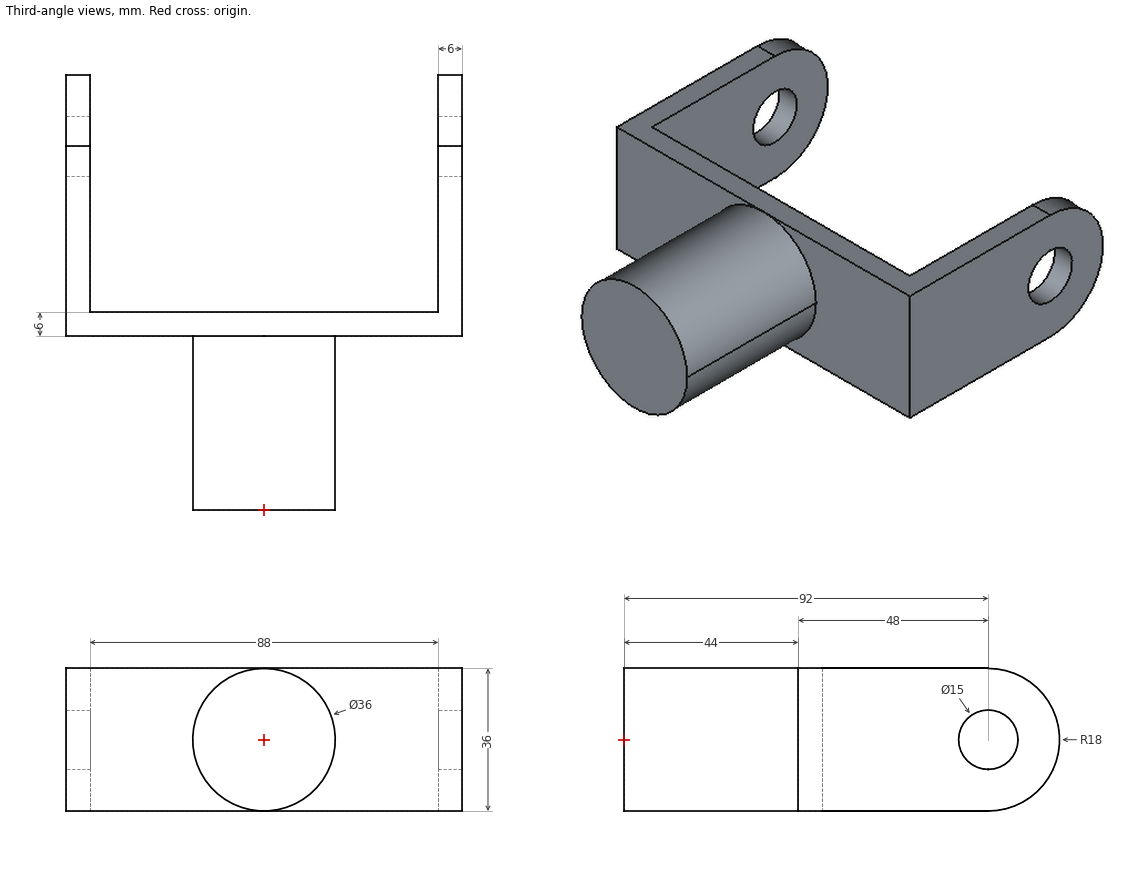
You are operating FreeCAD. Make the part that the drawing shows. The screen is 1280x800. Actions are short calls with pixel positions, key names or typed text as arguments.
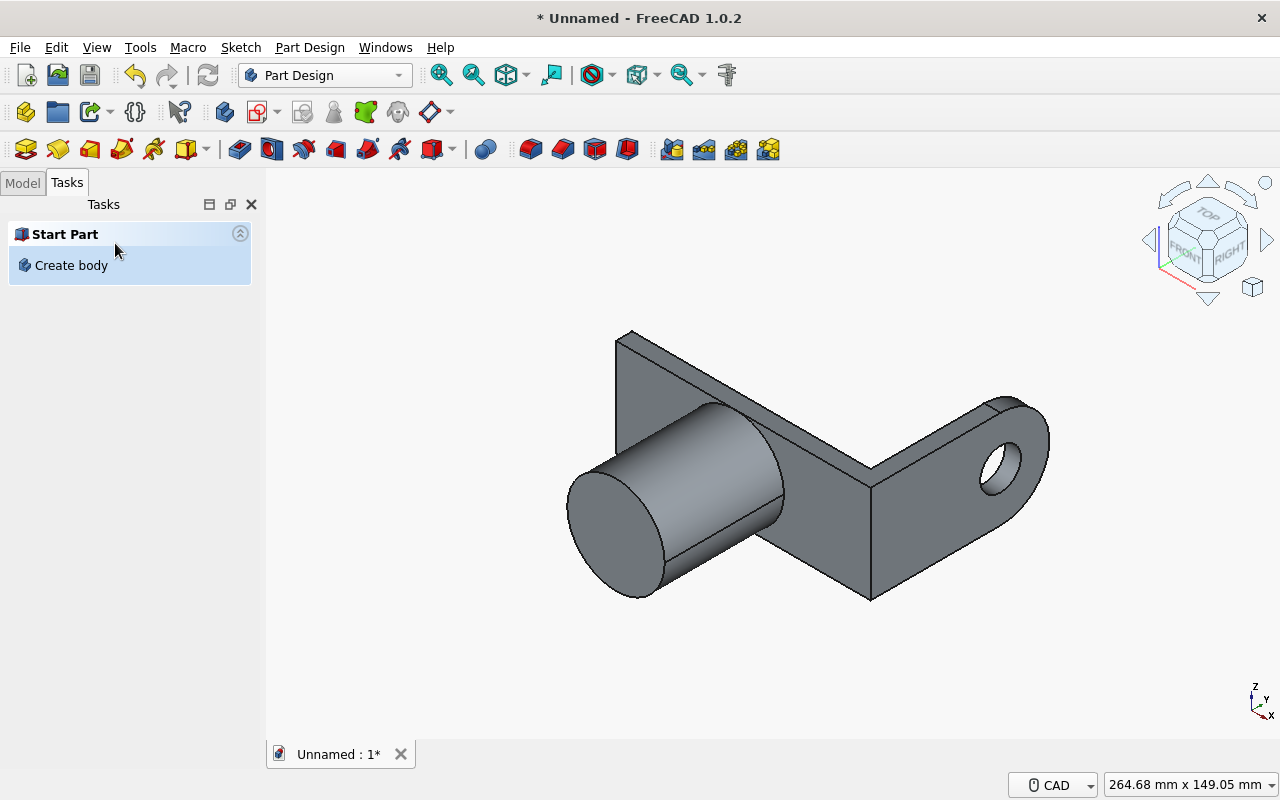
click(23, 182)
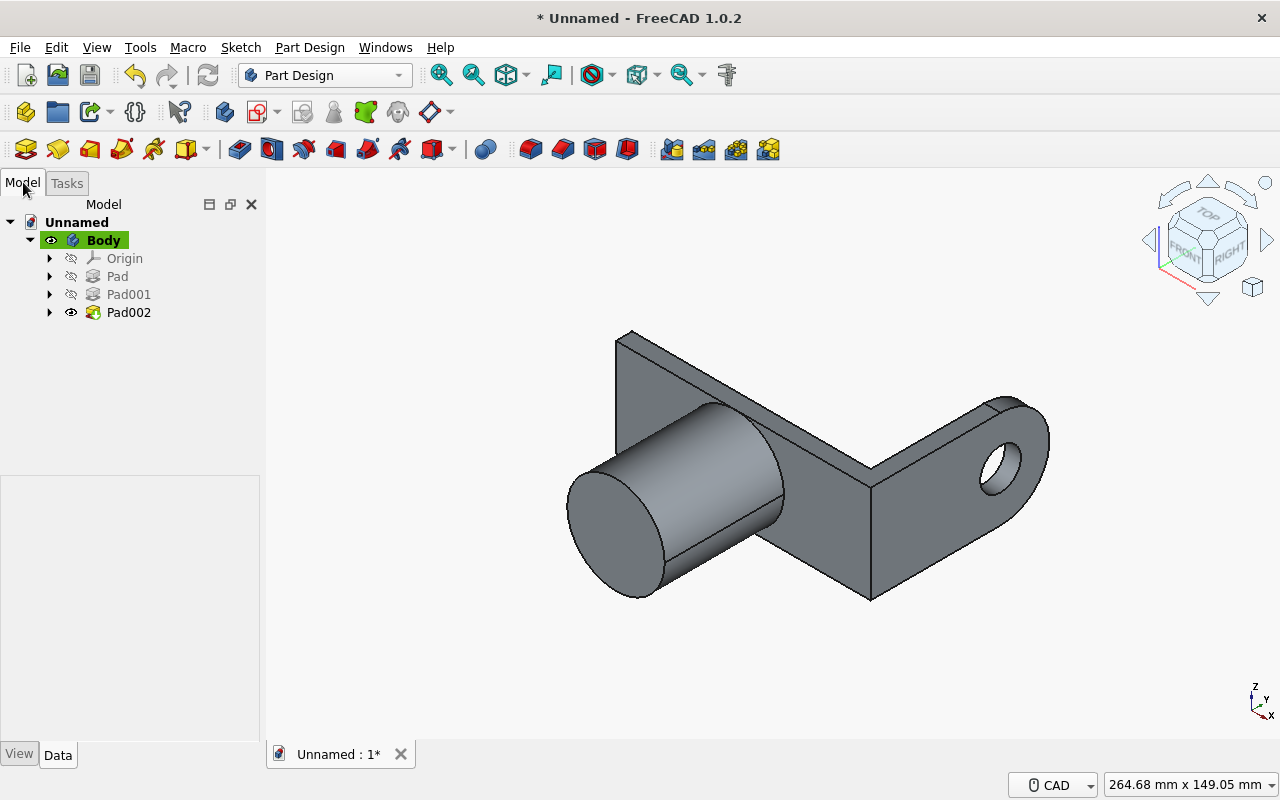
click(116, 312)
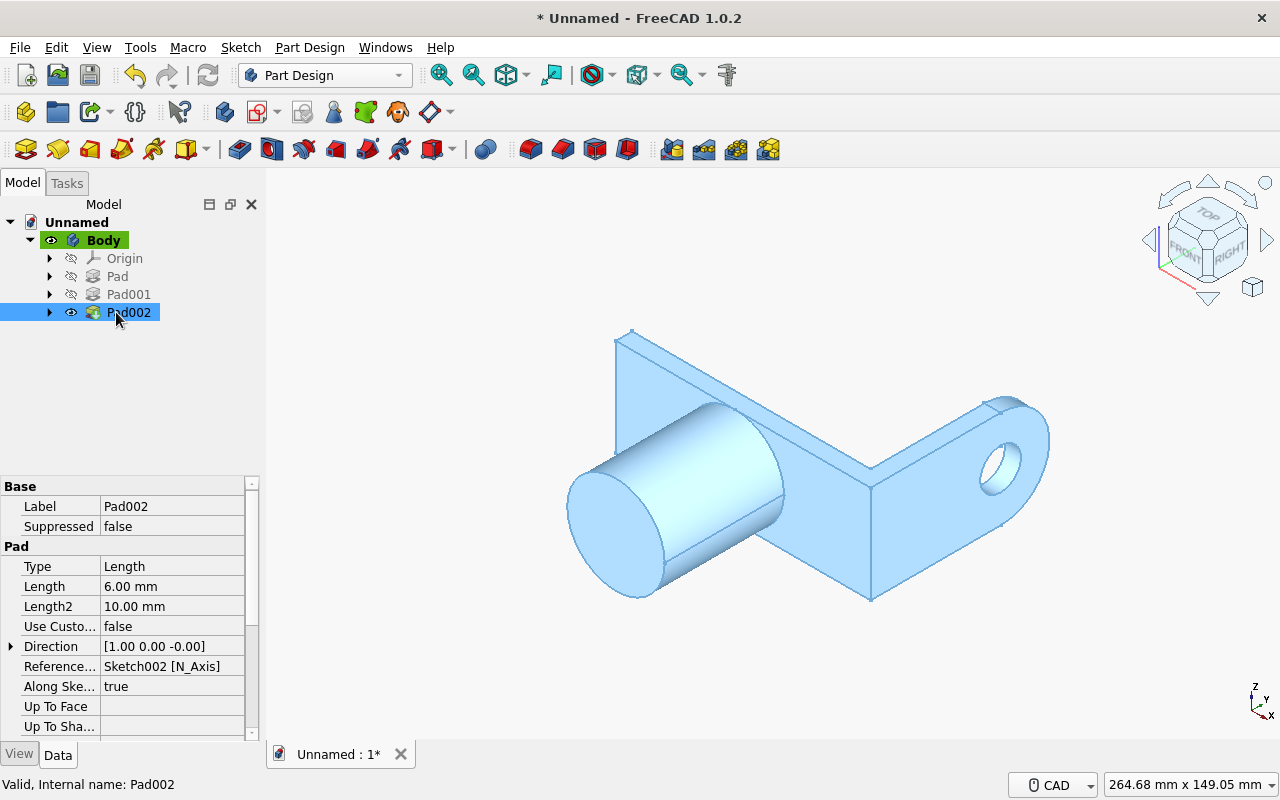
click(672, 150)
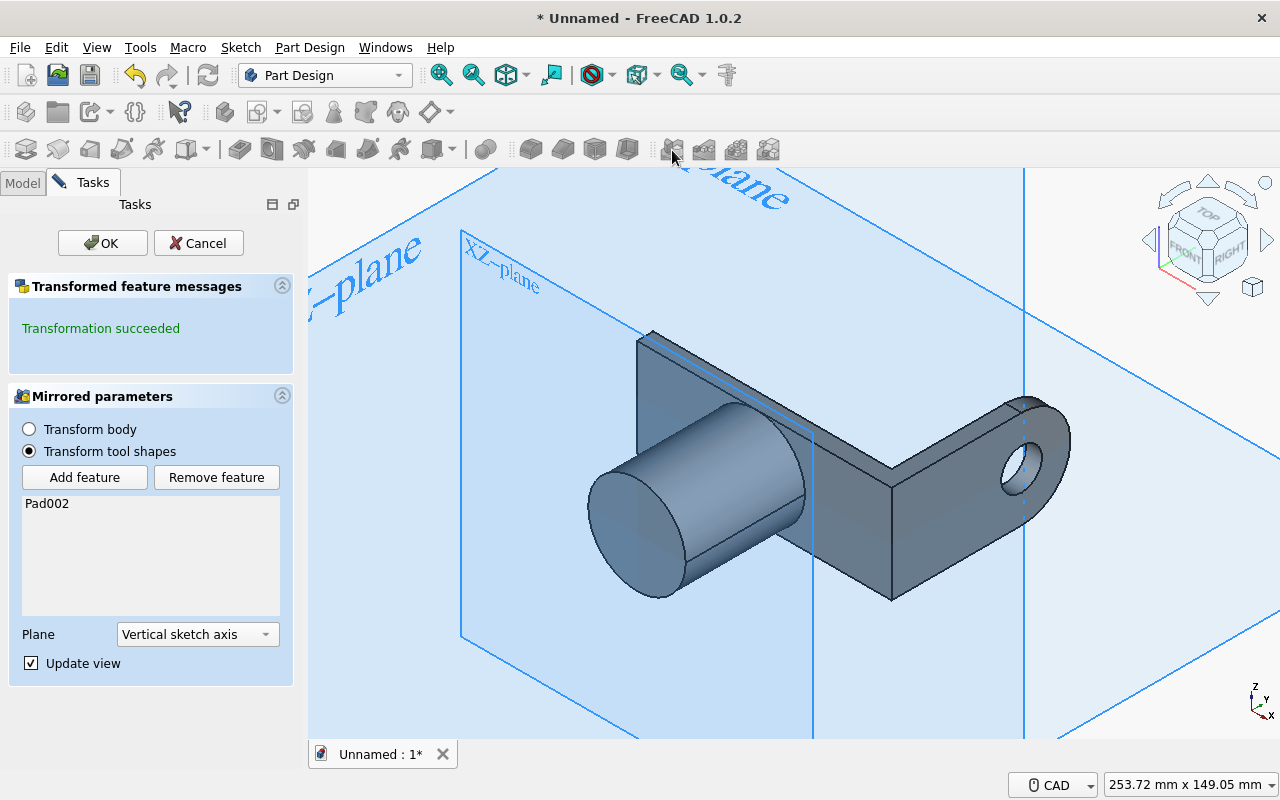
click(198, 634)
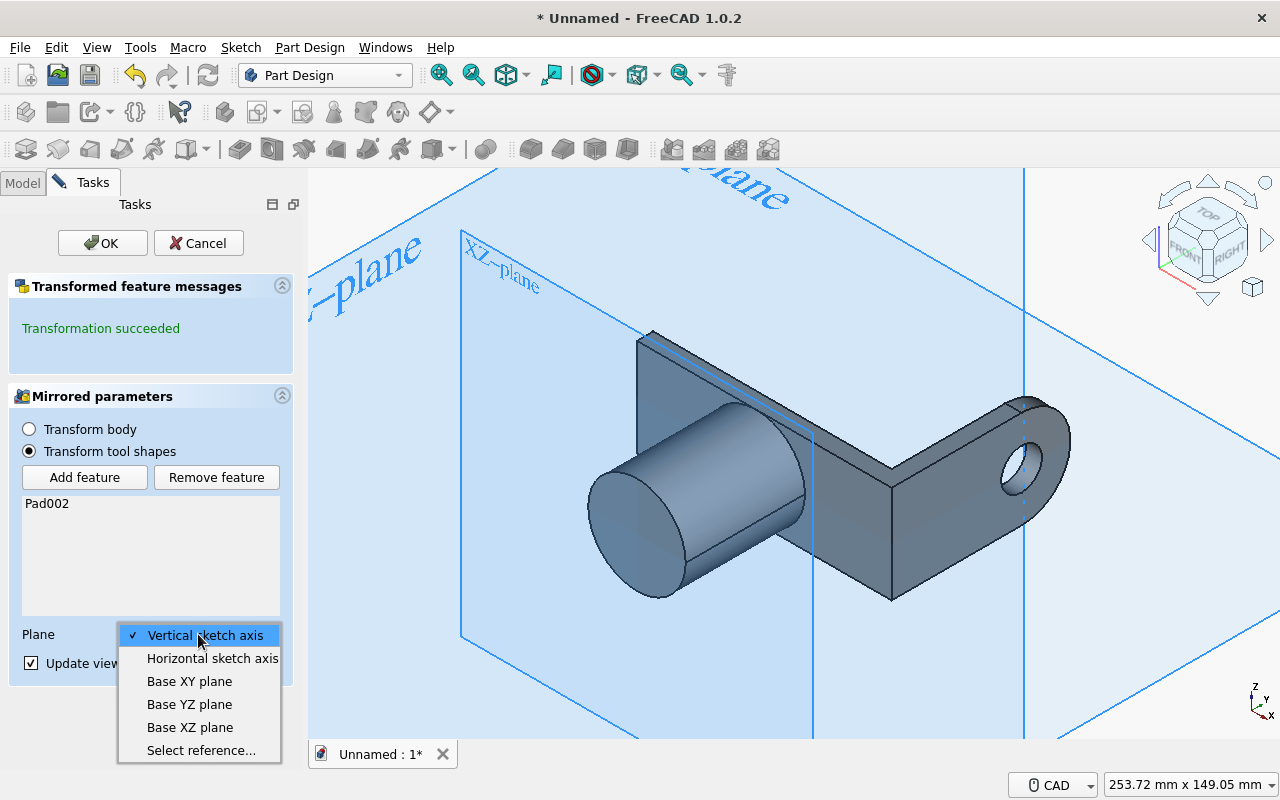
click(198, 704)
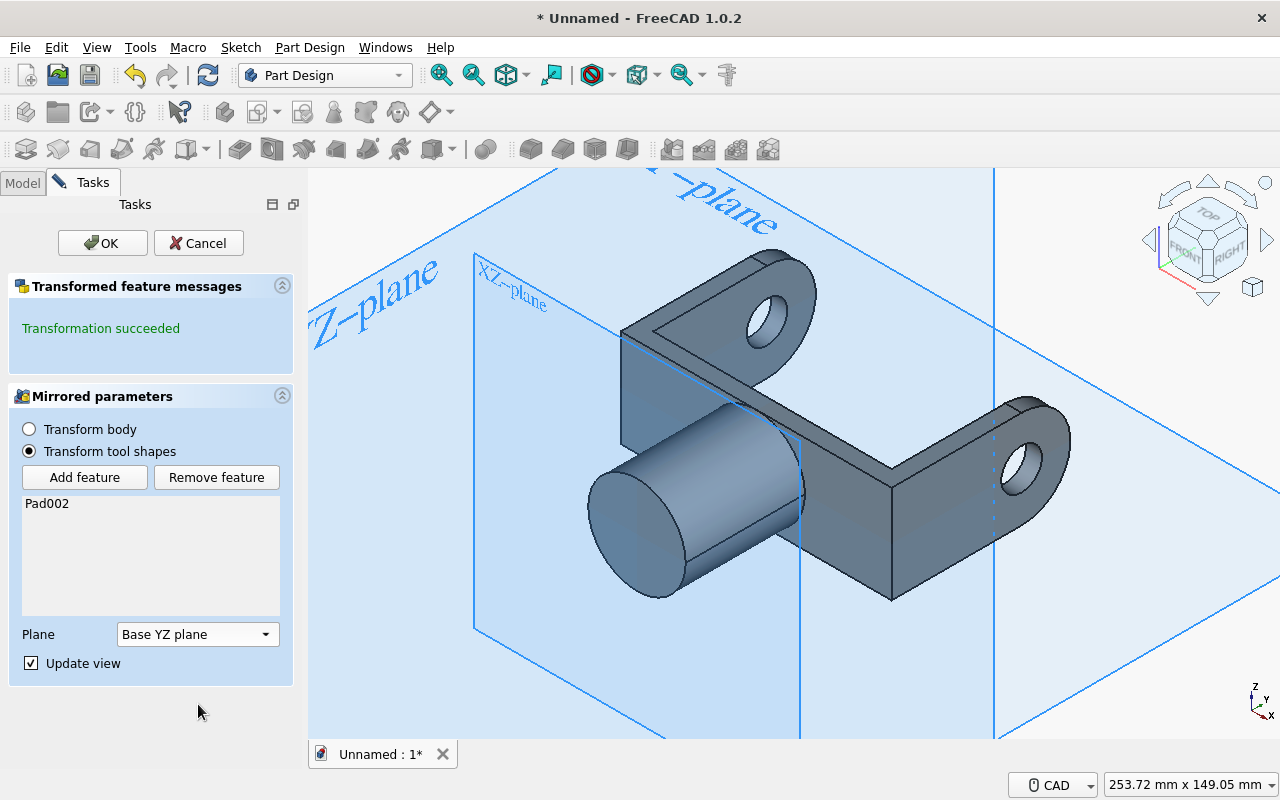
click(103, 243)